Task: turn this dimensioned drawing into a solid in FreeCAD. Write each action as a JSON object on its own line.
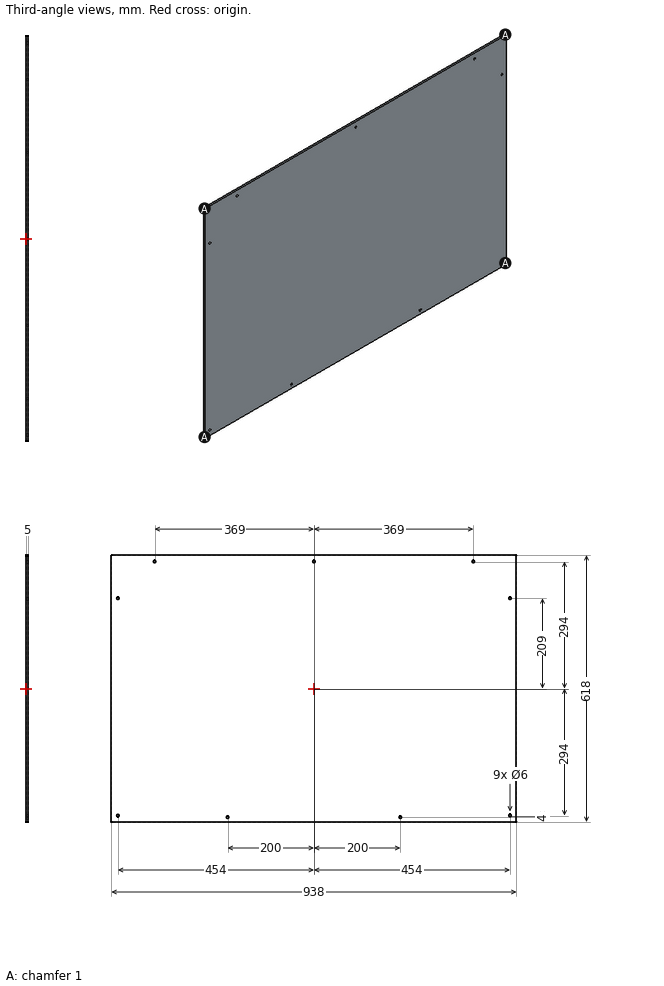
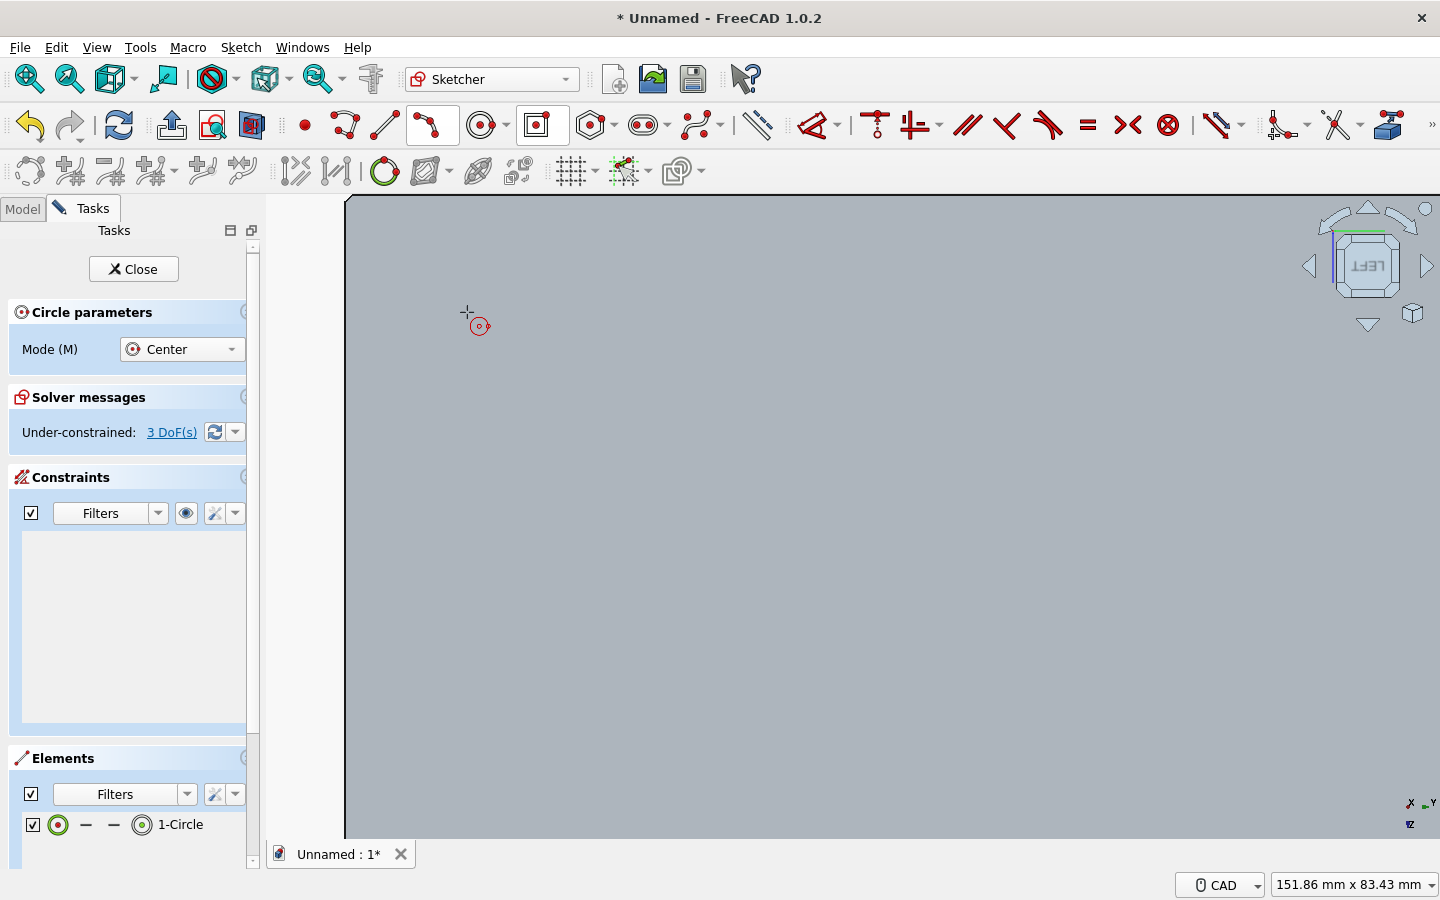
{"action": "scroll", "coordinate": [467, 312], "scroll_direction": "down", "scroll_amount": 12}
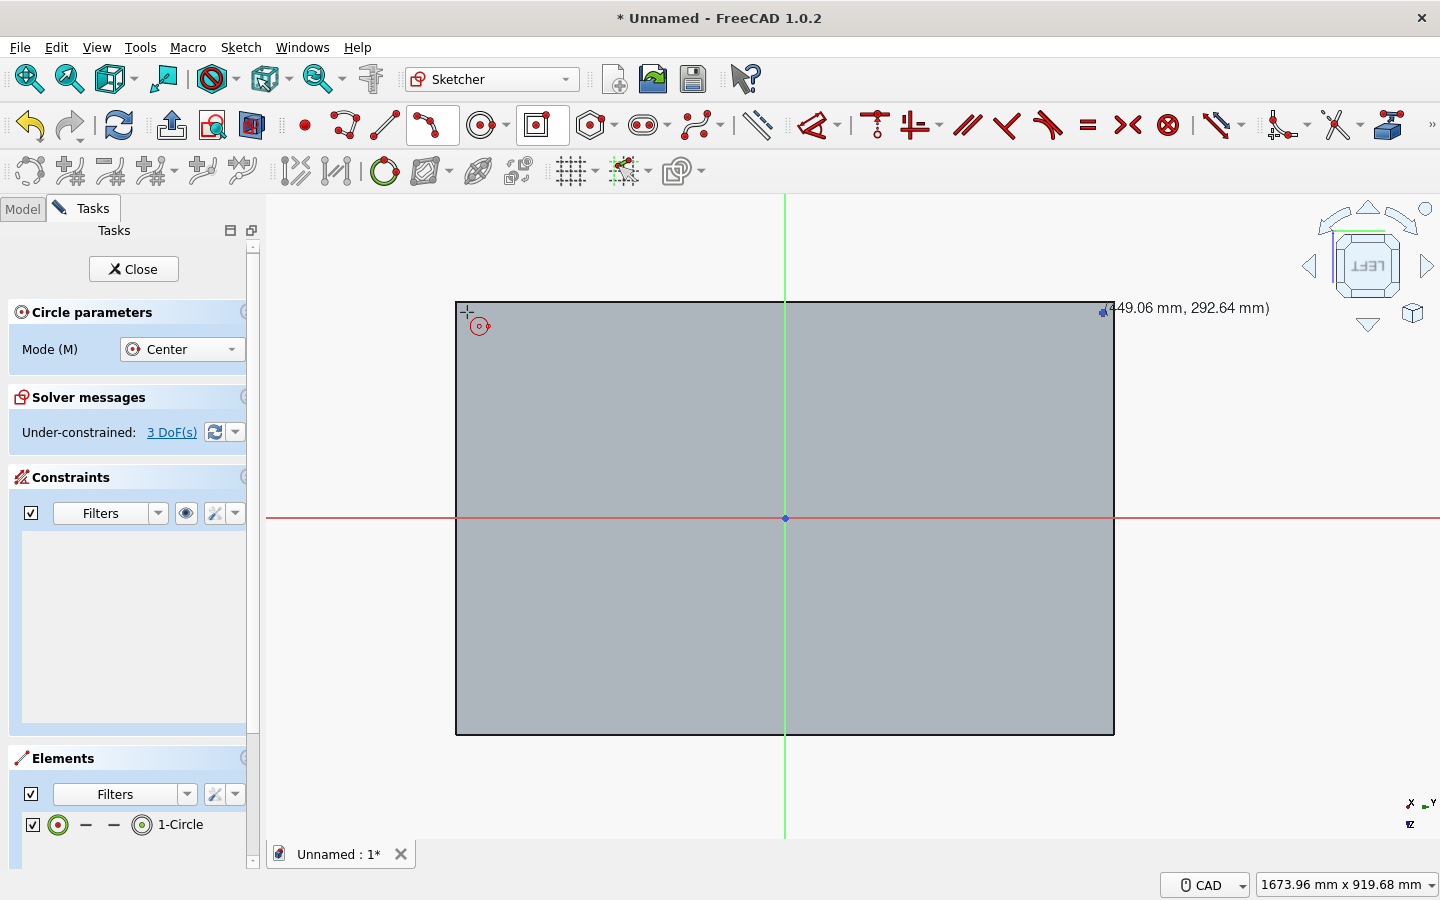
{"action": "left_click", "coordinate": [467, 312]}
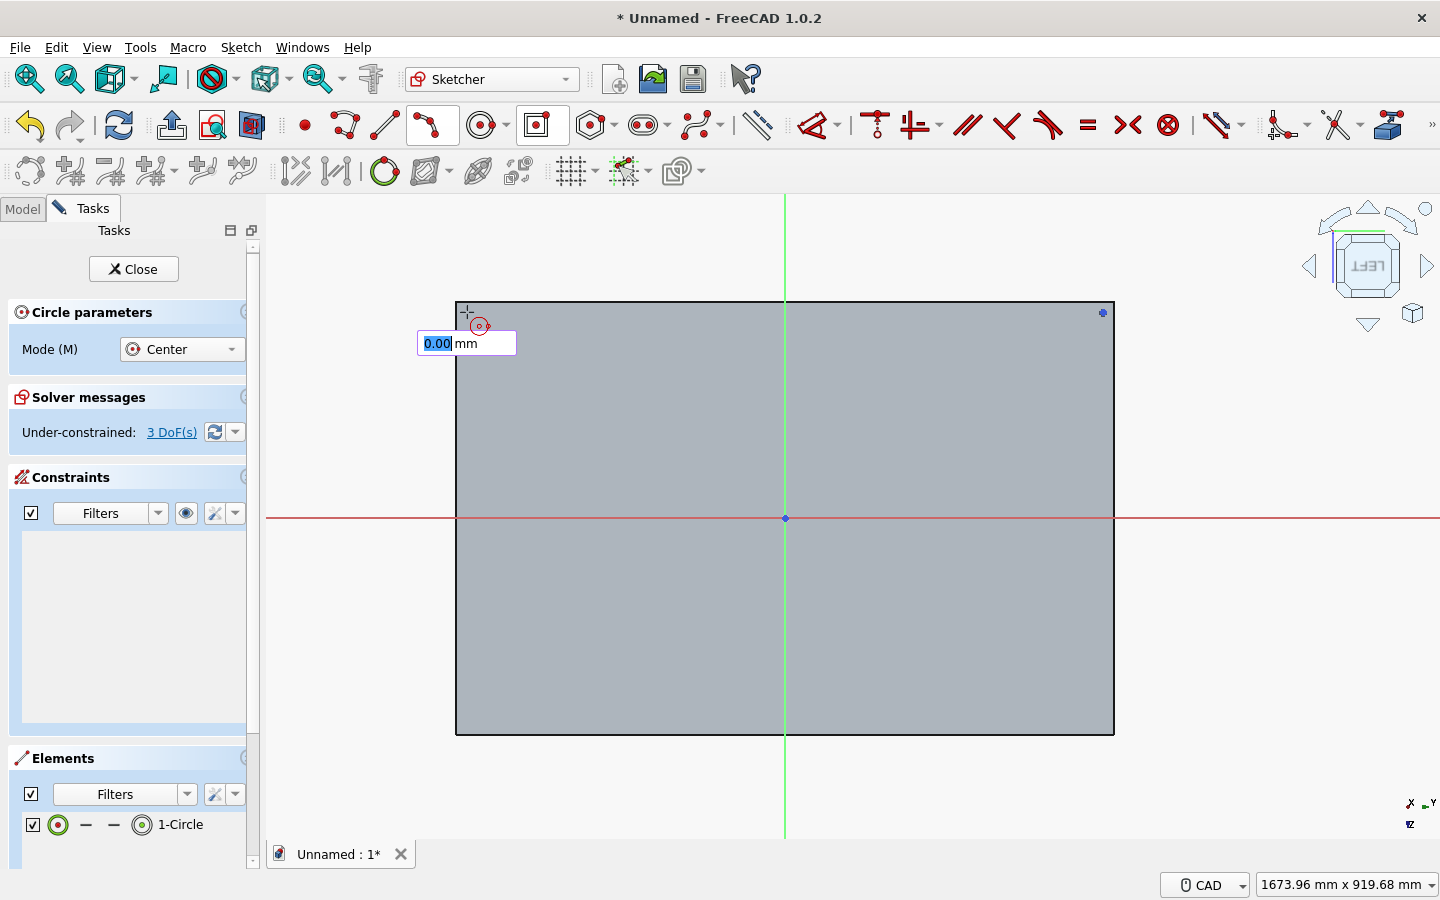
{"action": "scroll", "coordinate": [468, 311], "scroll_direction": "up", "scroll_amount": 11}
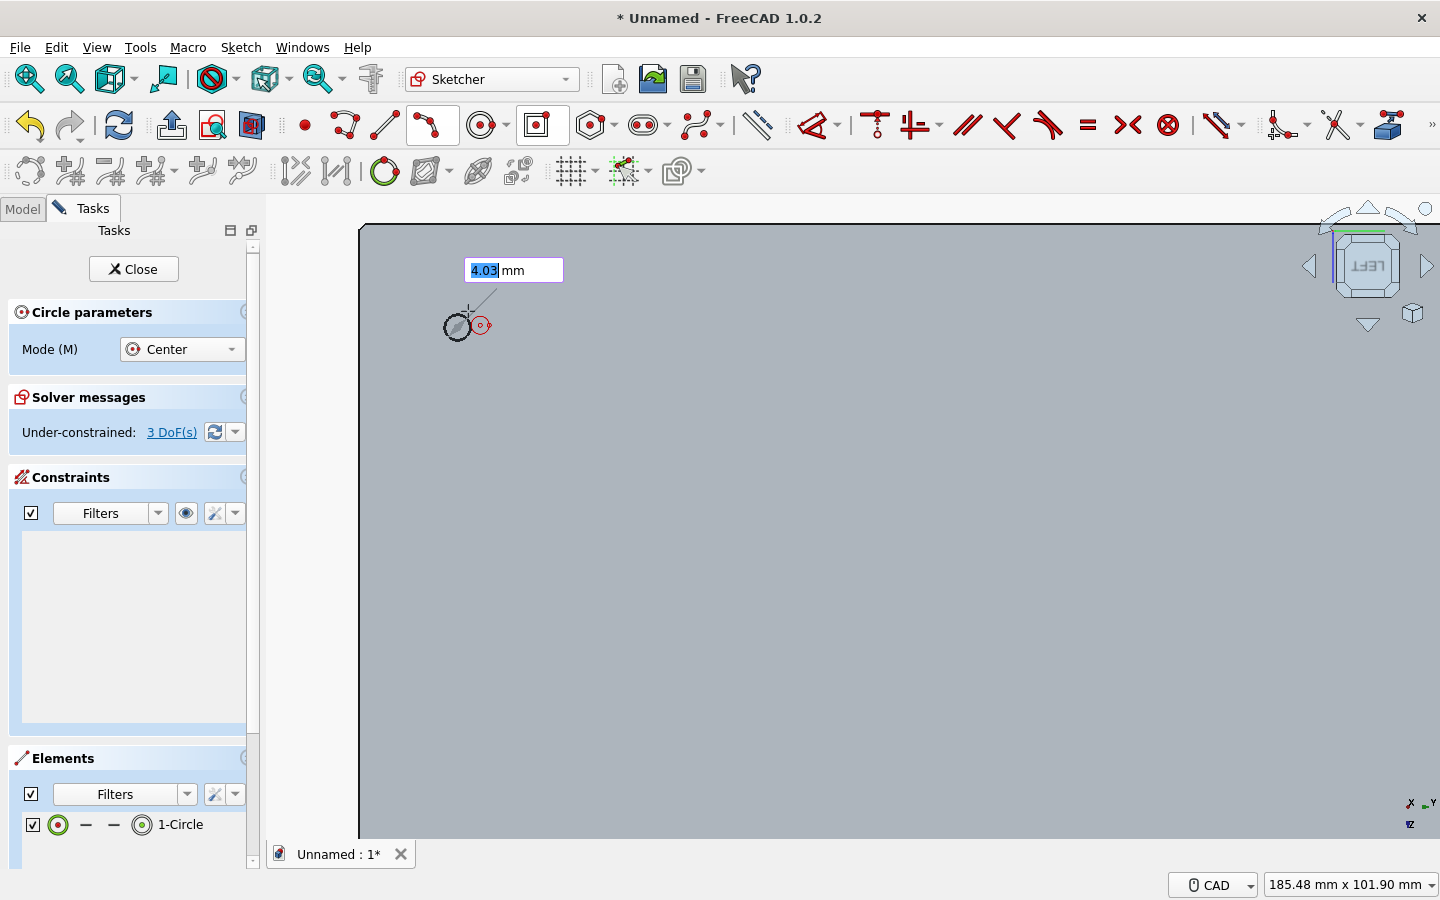
{"action": "left_click", "coordinate": [468, 306]}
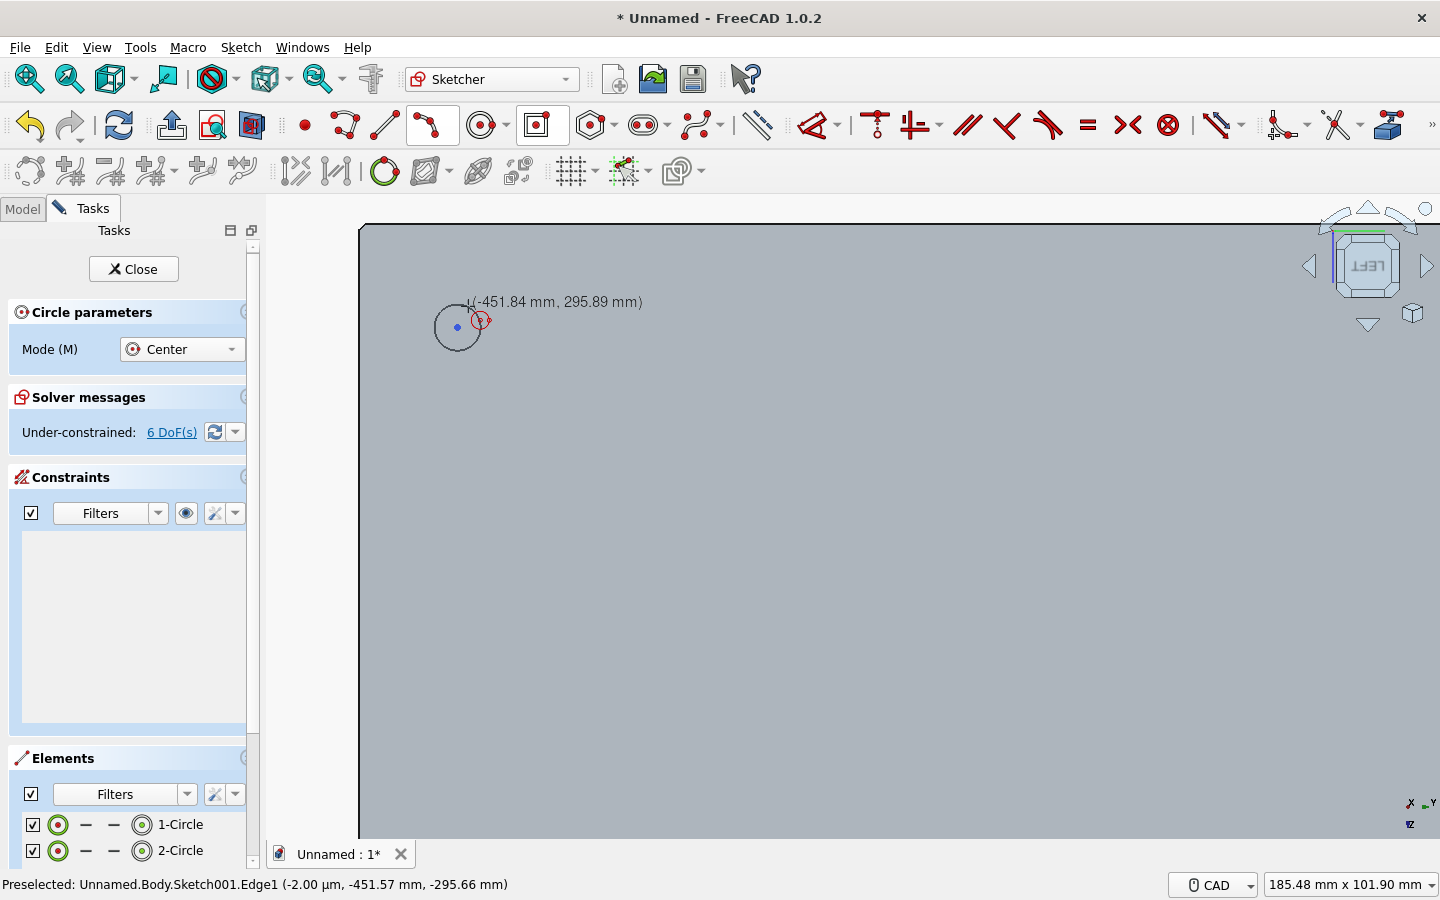
{"action": "scroll", "coordinate": [468, 311], "scroll_direction": "down", "scroll_amount": 11}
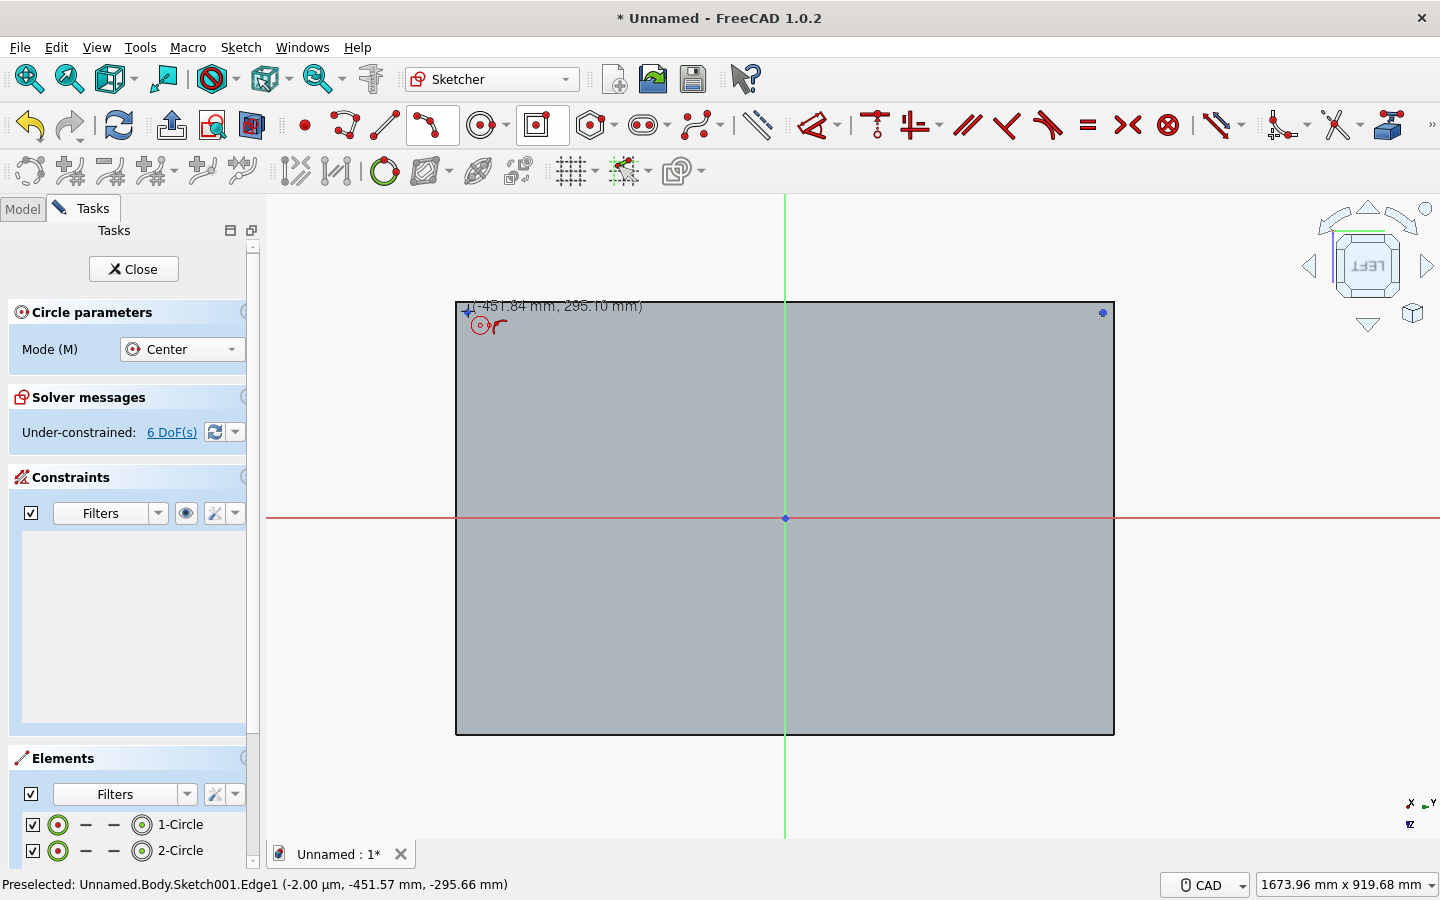
{"action": "scroll", "coordinate": [1103, 665], "scroll_direction": "up", "scroll_amount": 12}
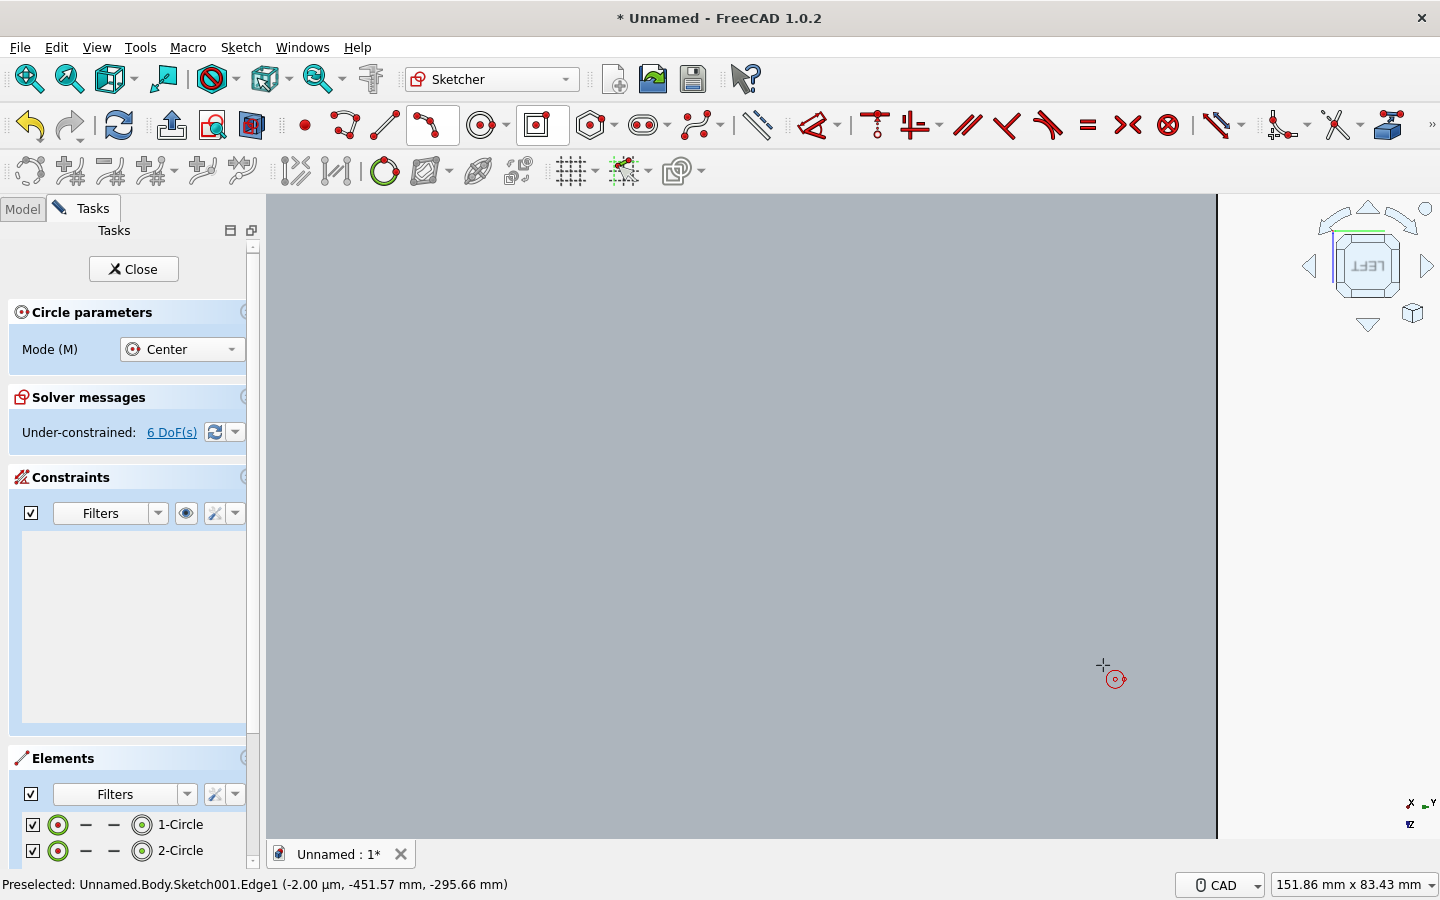
{"action": "scroll", "coordinate": [1103, 665], "scroll_direction": "down", "scroll_amount": 12}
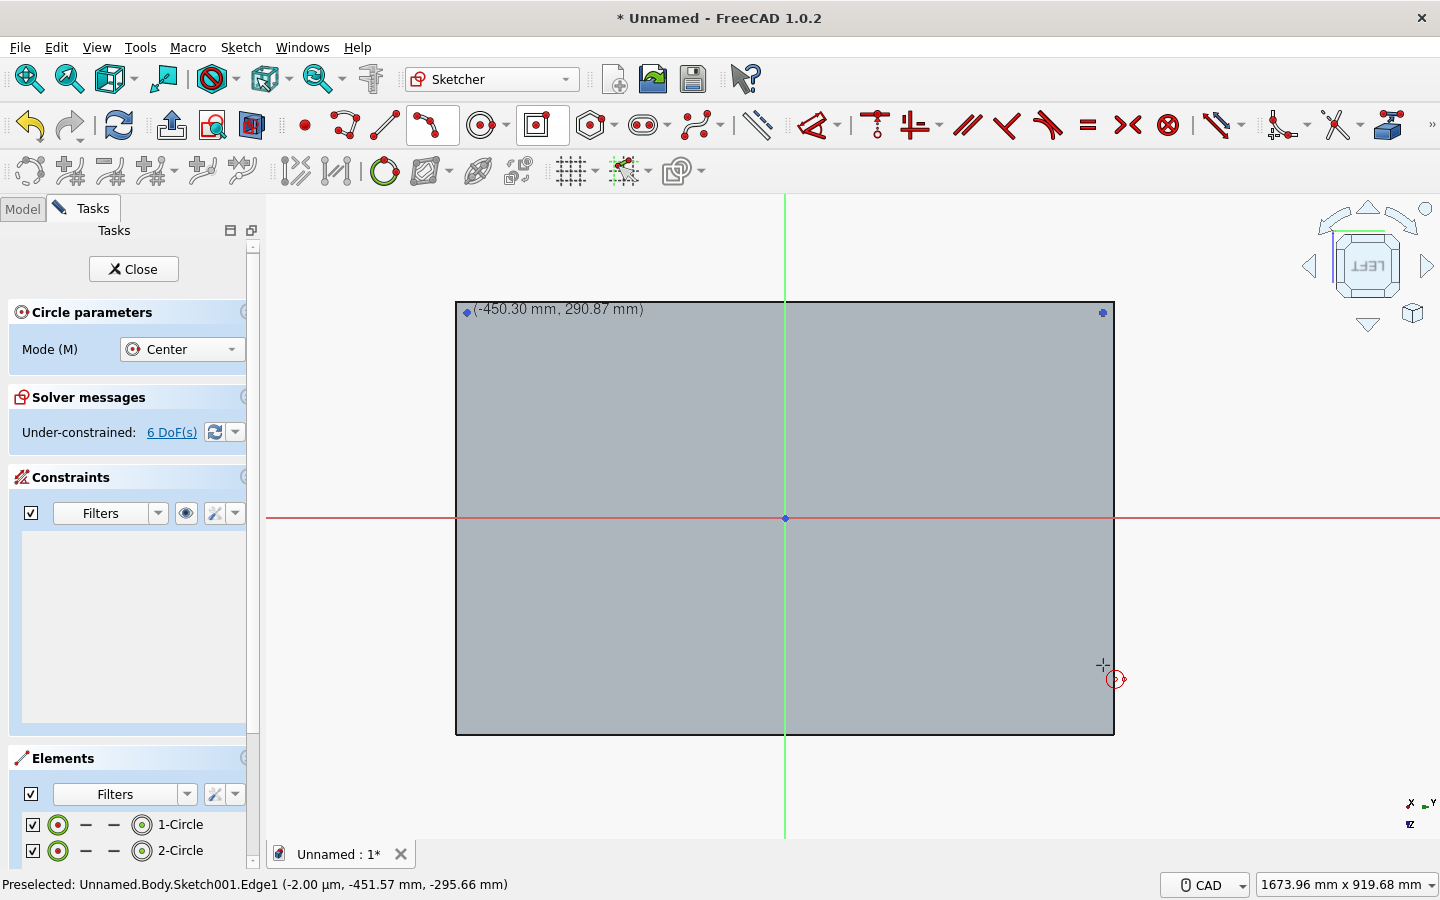
{"action": "left_click", "coordinate": [1103, 665]}